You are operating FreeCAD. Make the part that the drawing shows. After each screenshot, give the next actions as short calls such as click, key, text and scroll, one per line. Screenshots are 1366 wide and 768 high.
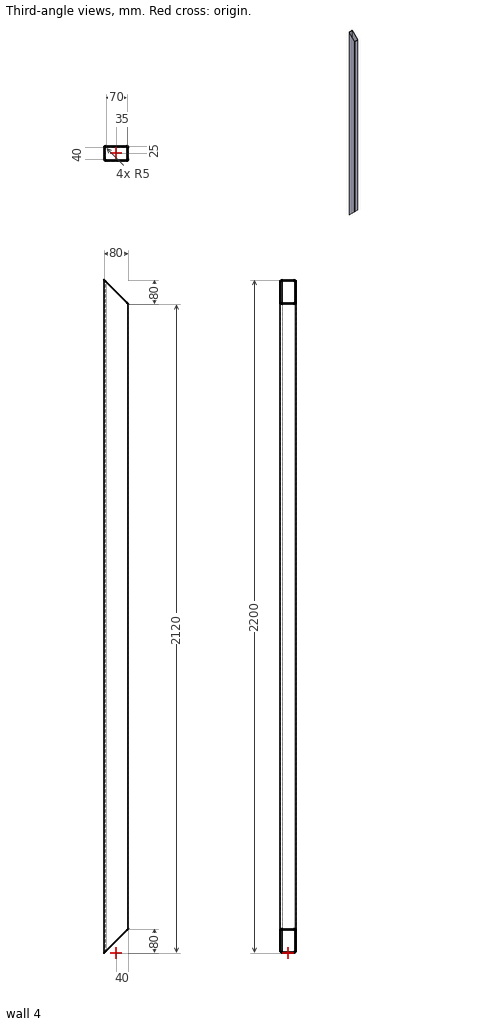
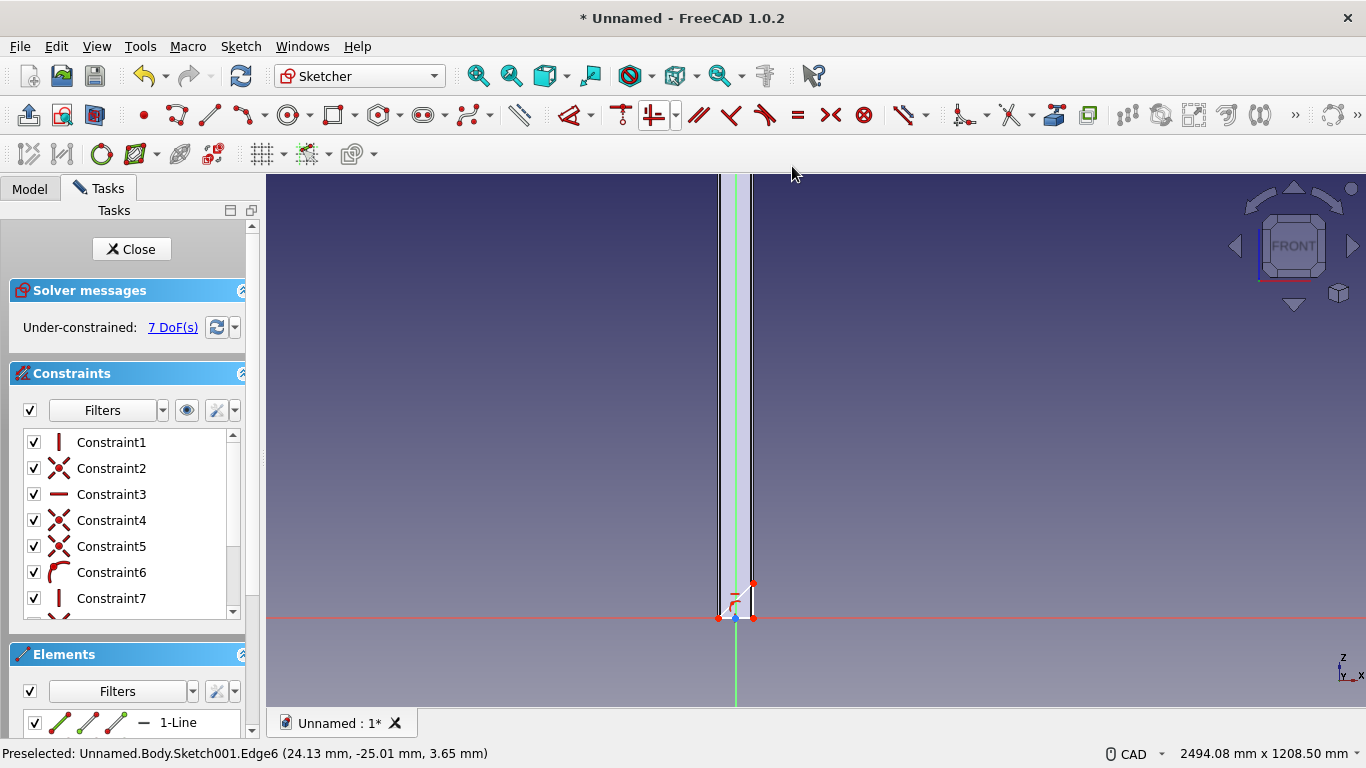
click(568, 116)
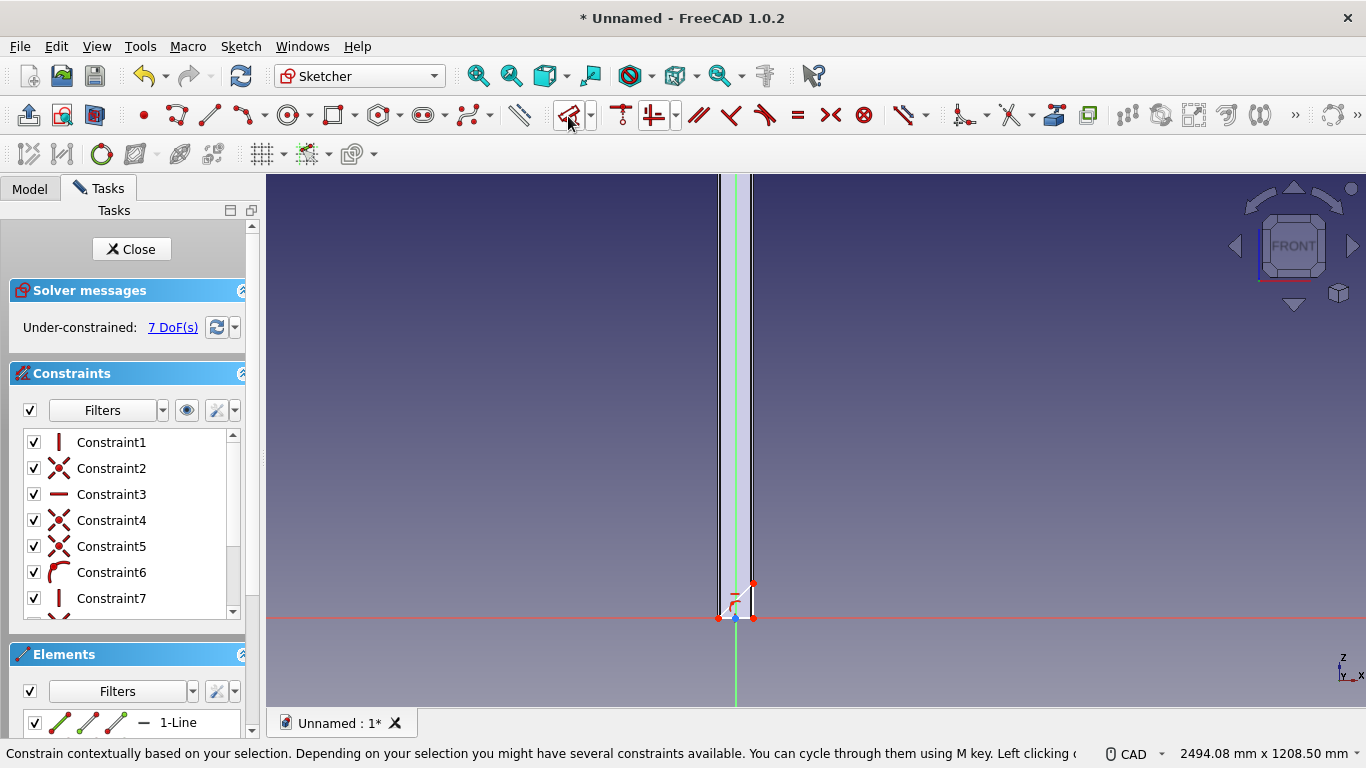
scroll(754, 619, down, 5)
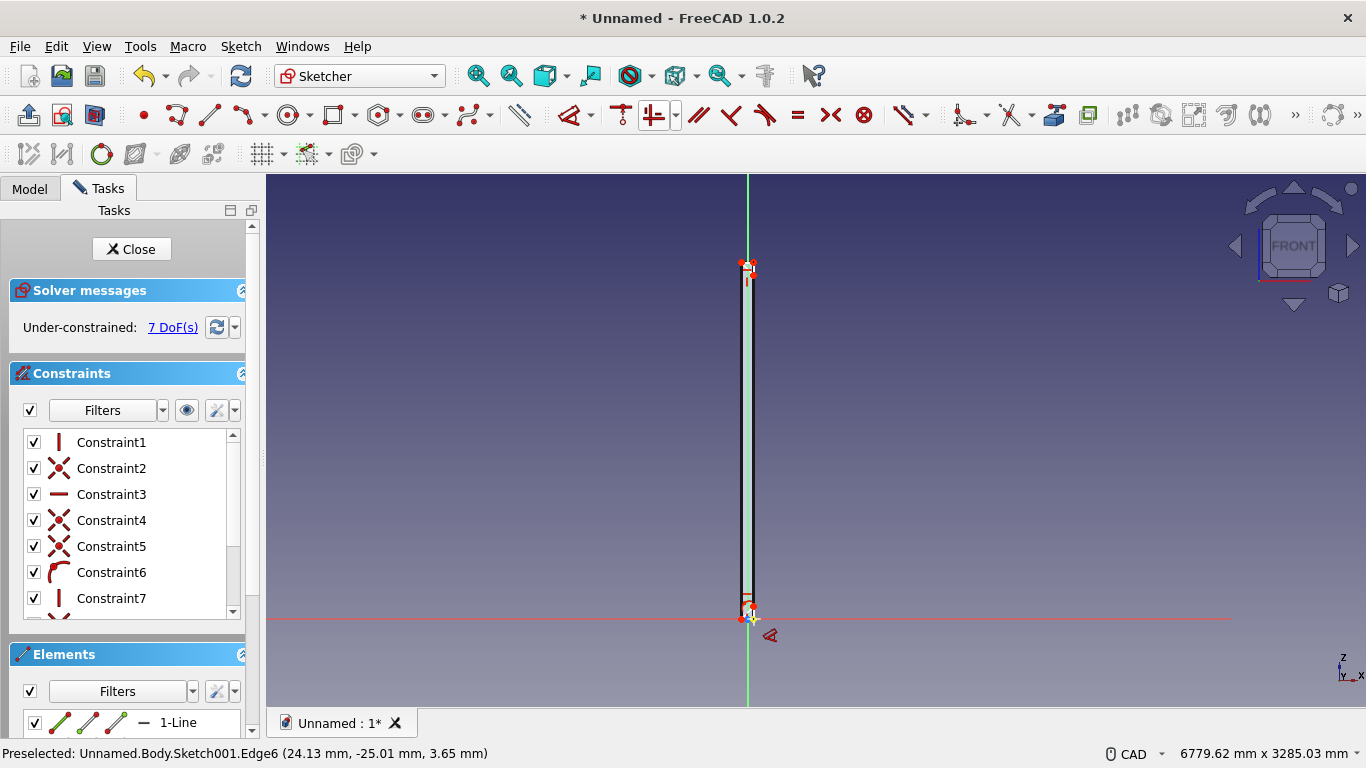
scroll(754, 267, up, 7)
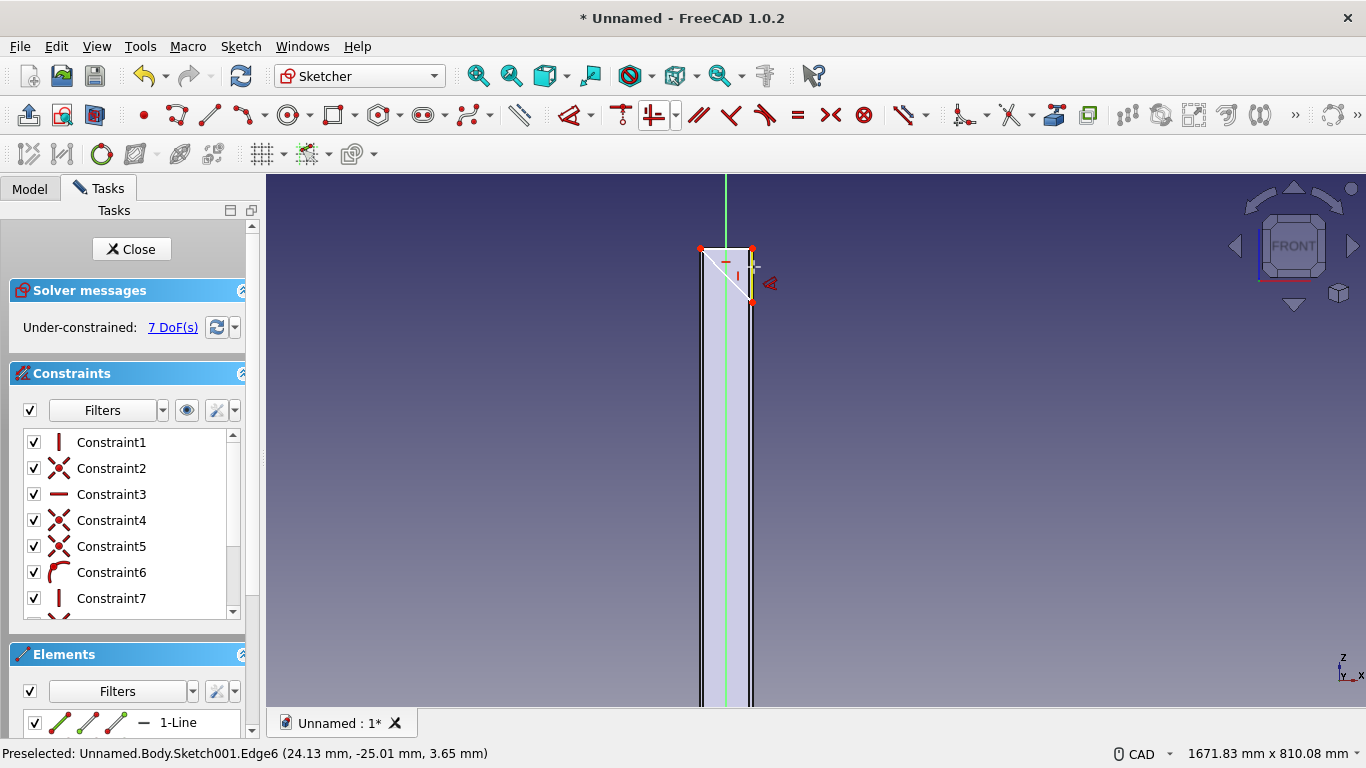
click(752, 265)
click(786, 276)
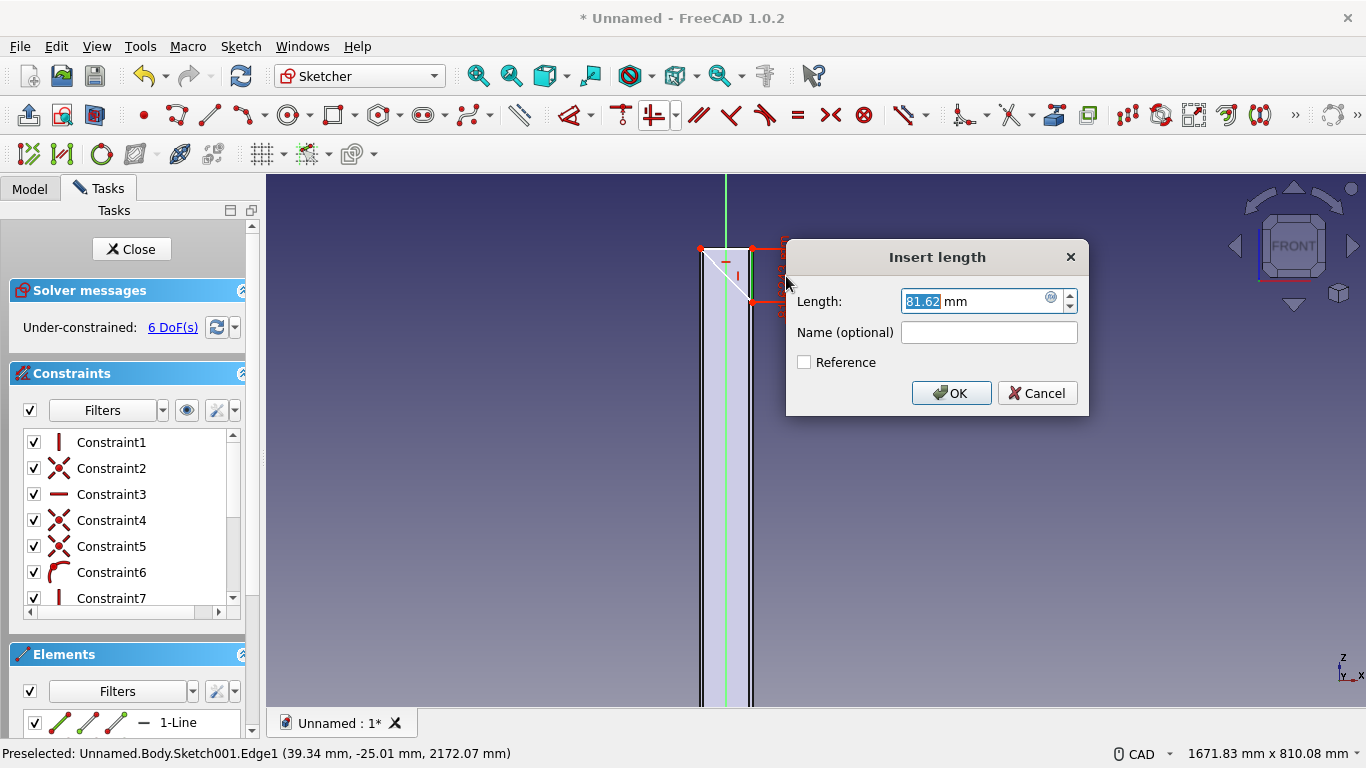
text(80)
key(Return)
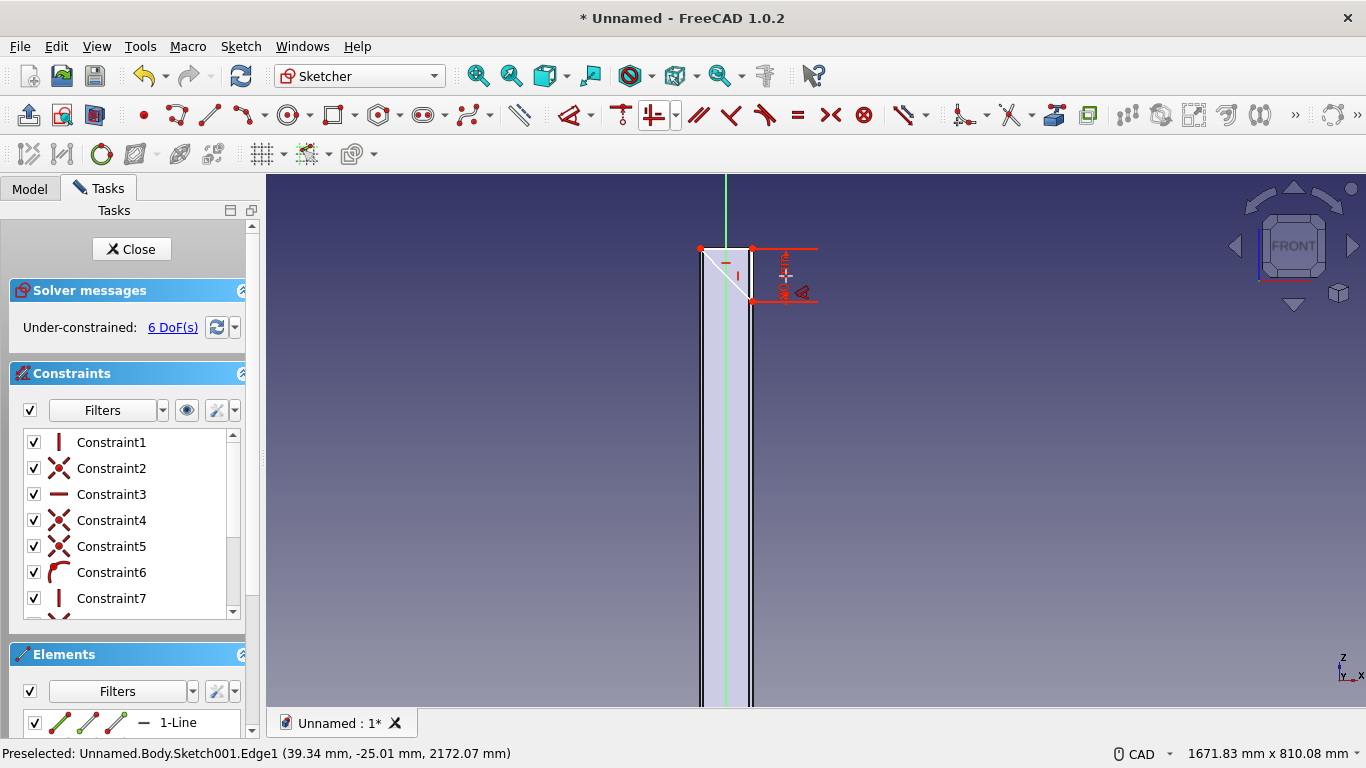
scroll(737, 249, up, 2)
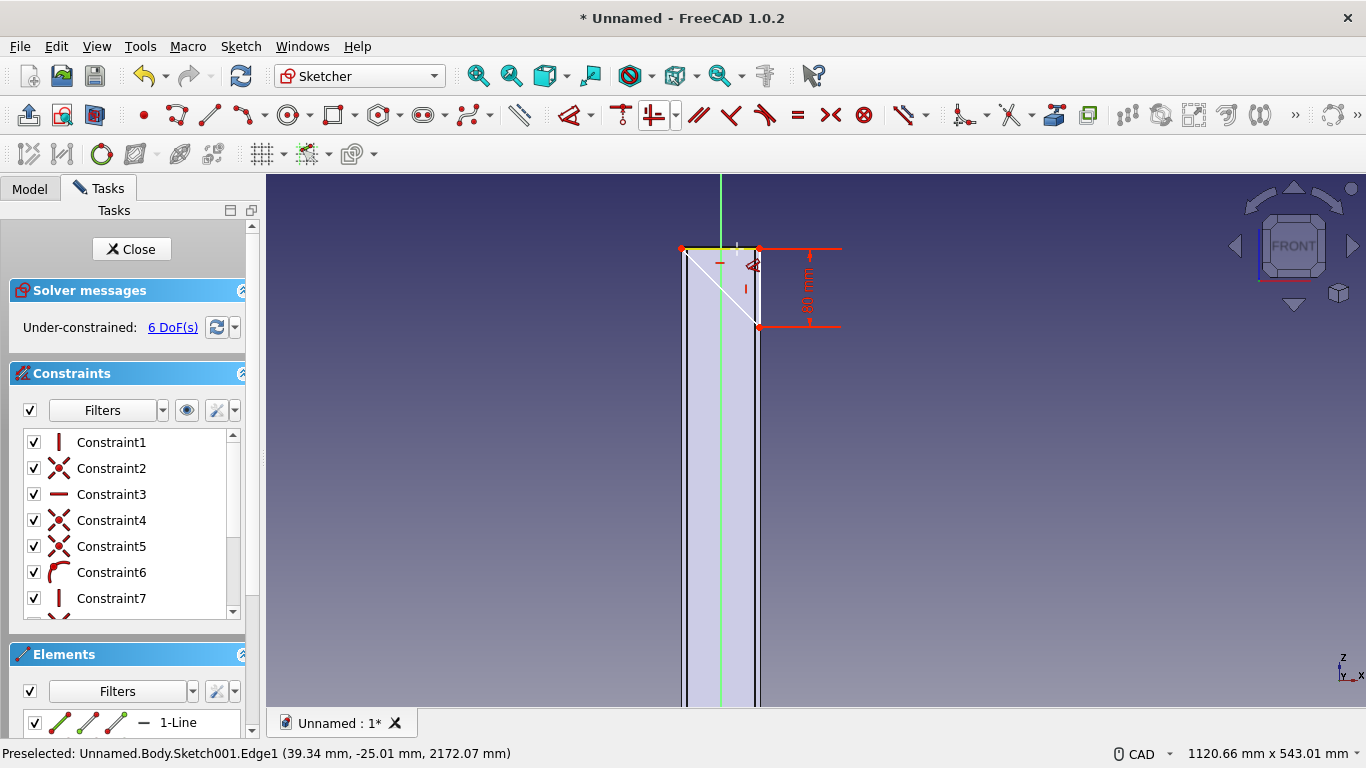
click(736, 249)
click(703, 215)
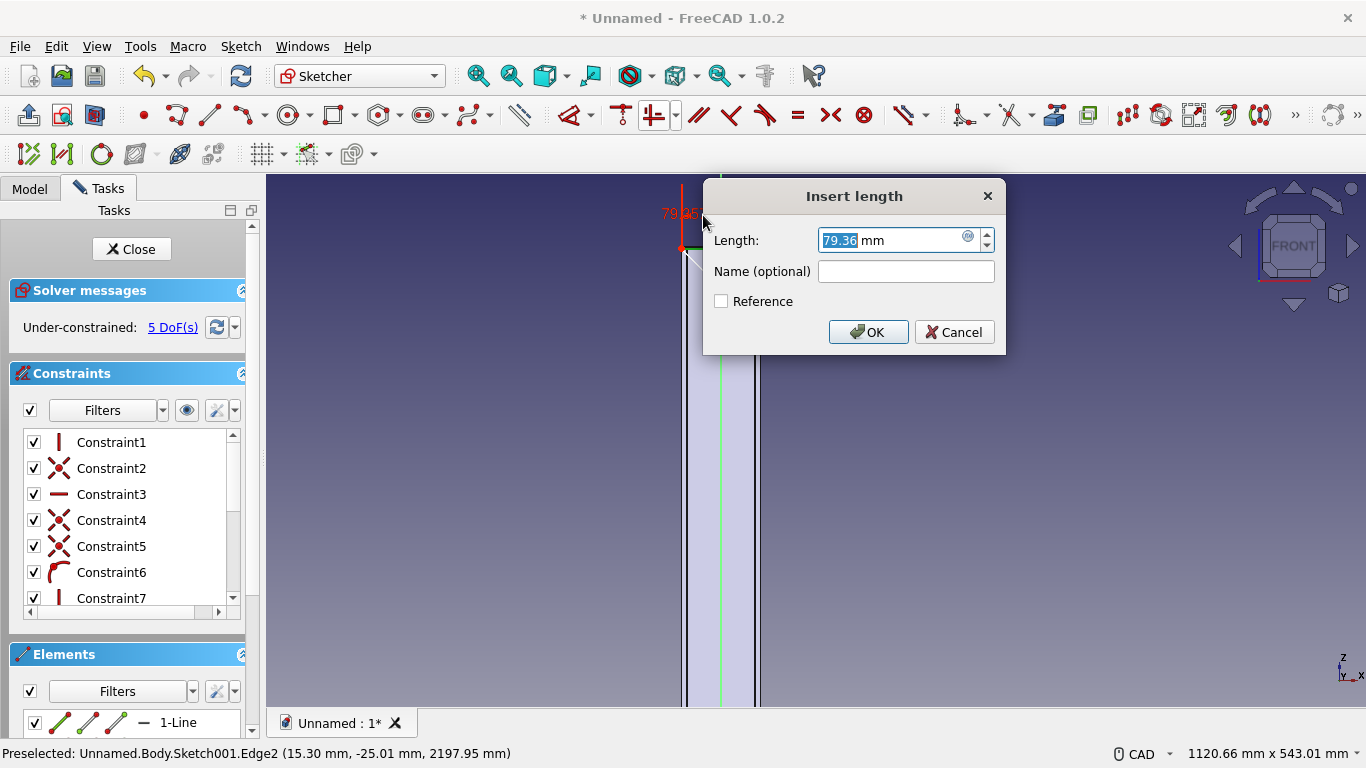
text(80)
key(Return)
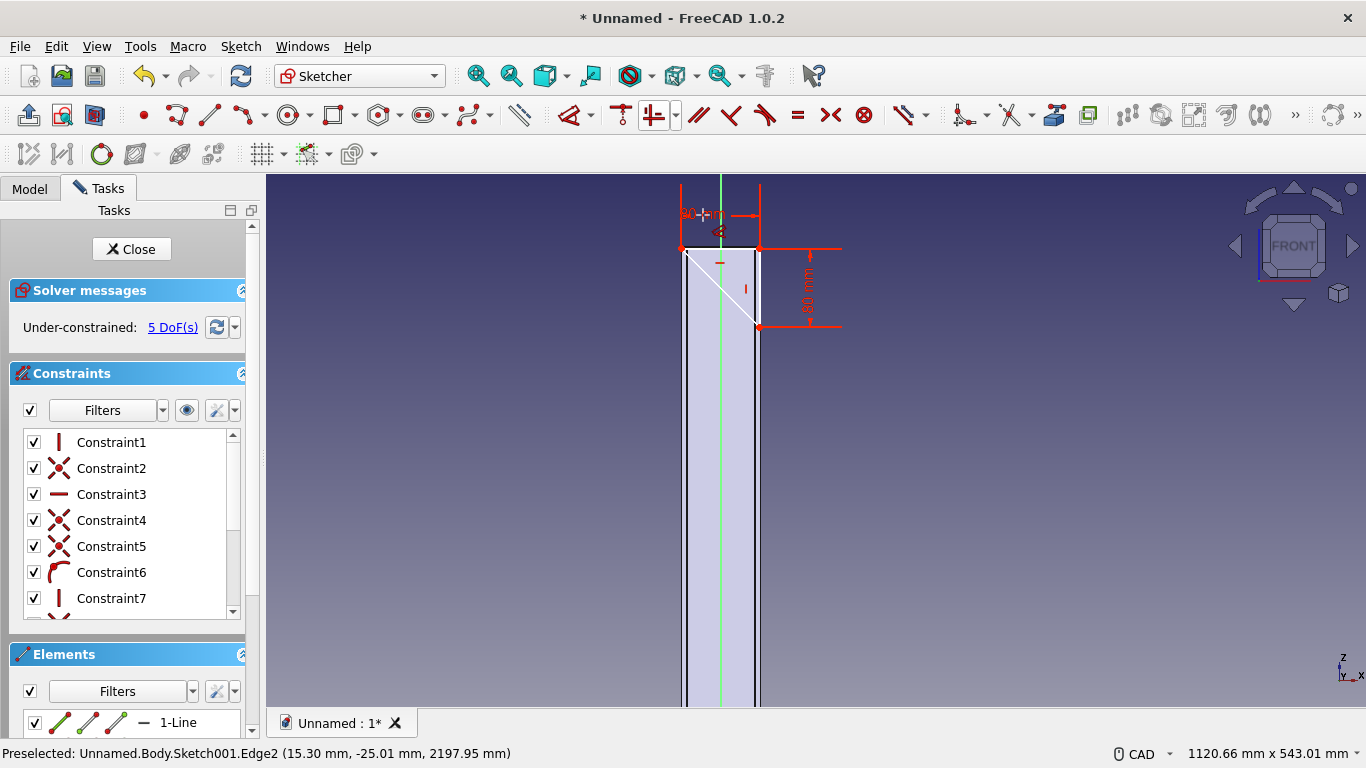
scroll(753, 265, down, 9)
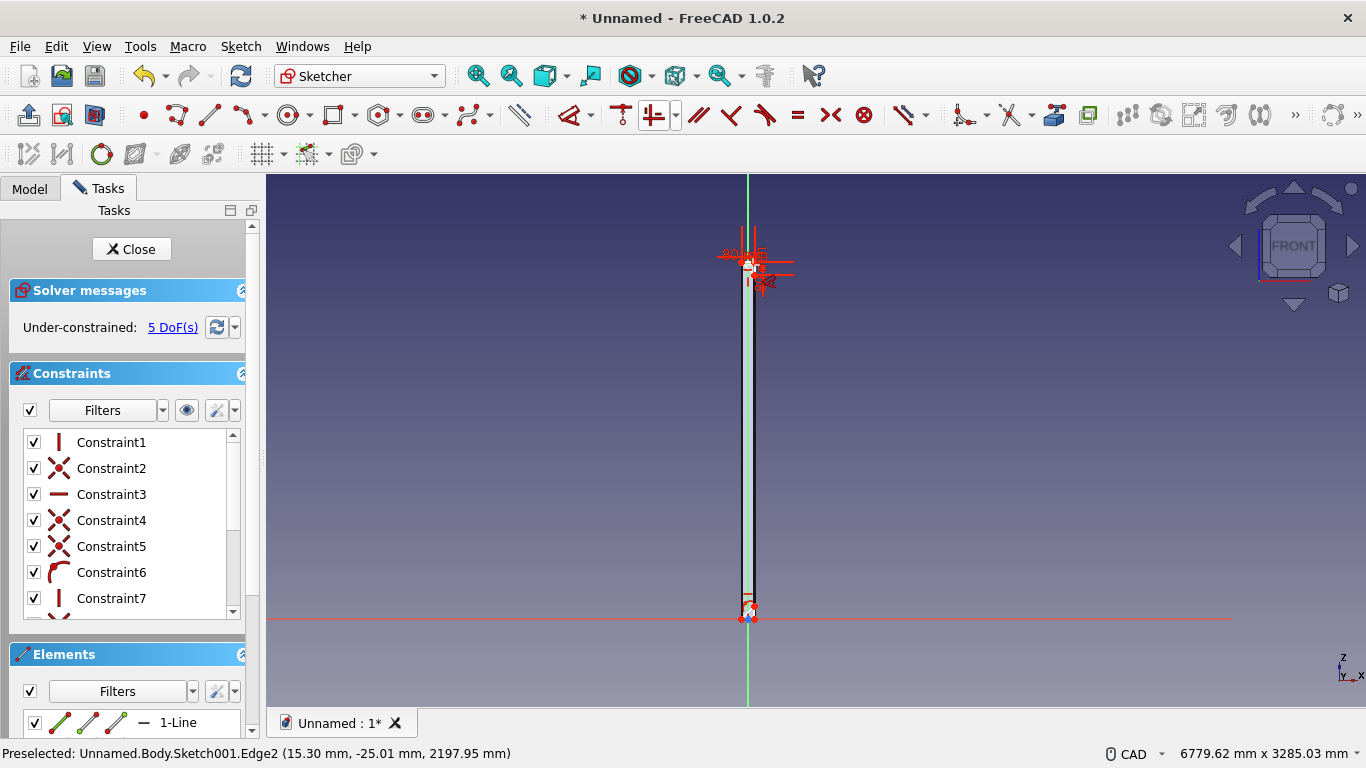
scroll(754, 615, up, 7)